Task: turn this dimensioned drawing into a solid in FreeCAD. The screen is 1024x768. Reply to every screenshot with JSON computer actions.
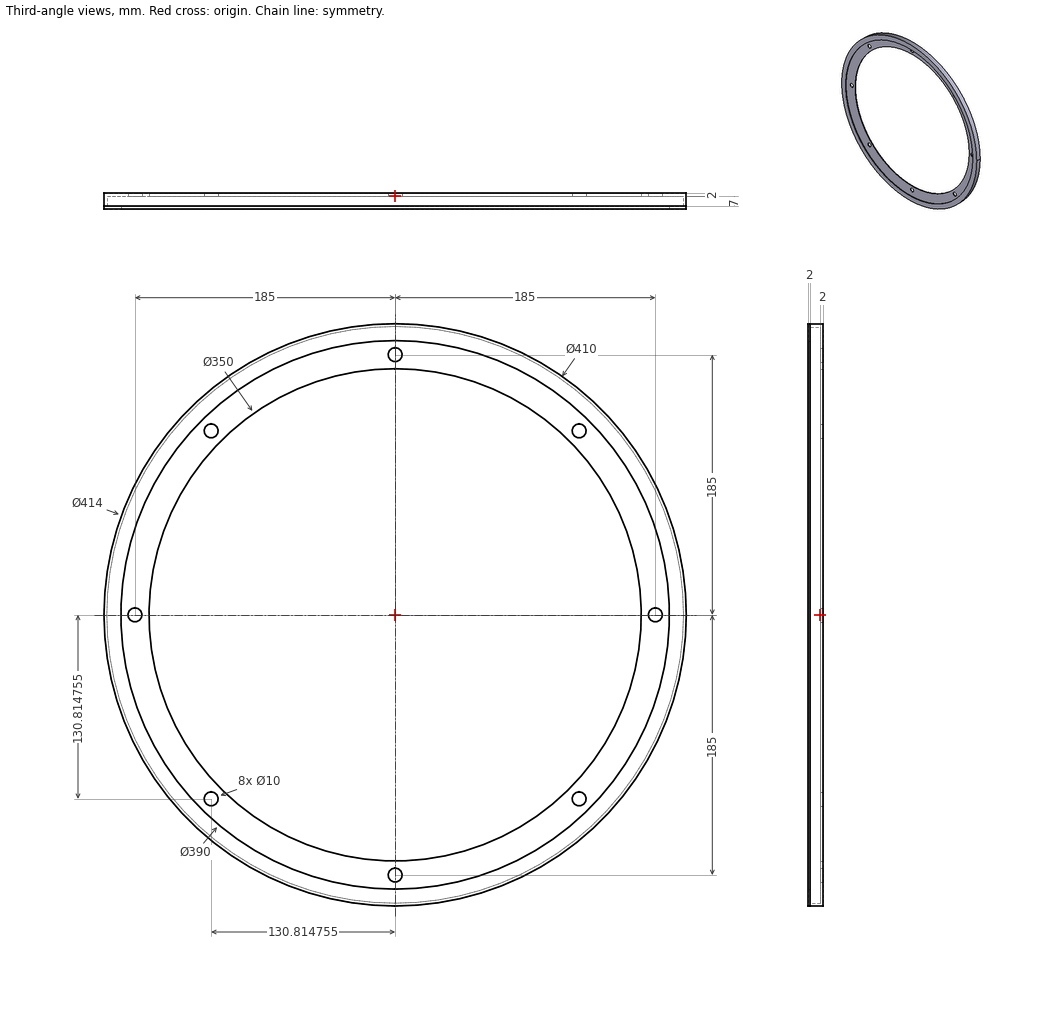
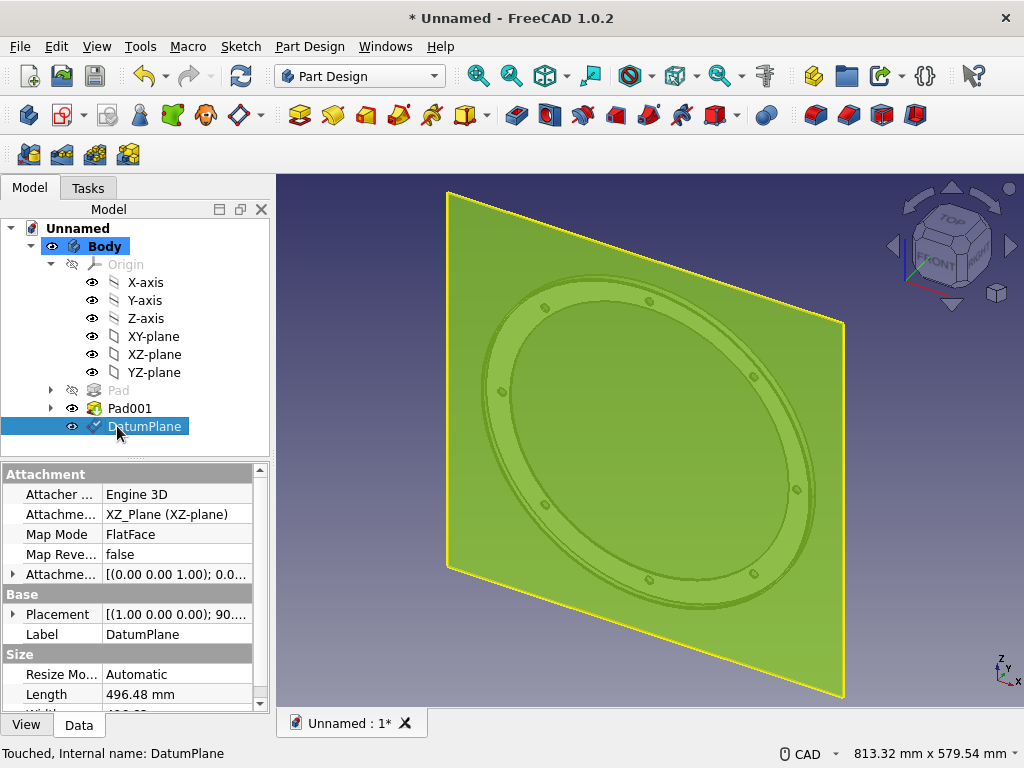
{"action": "left_click", "coordinate": [62, 116]}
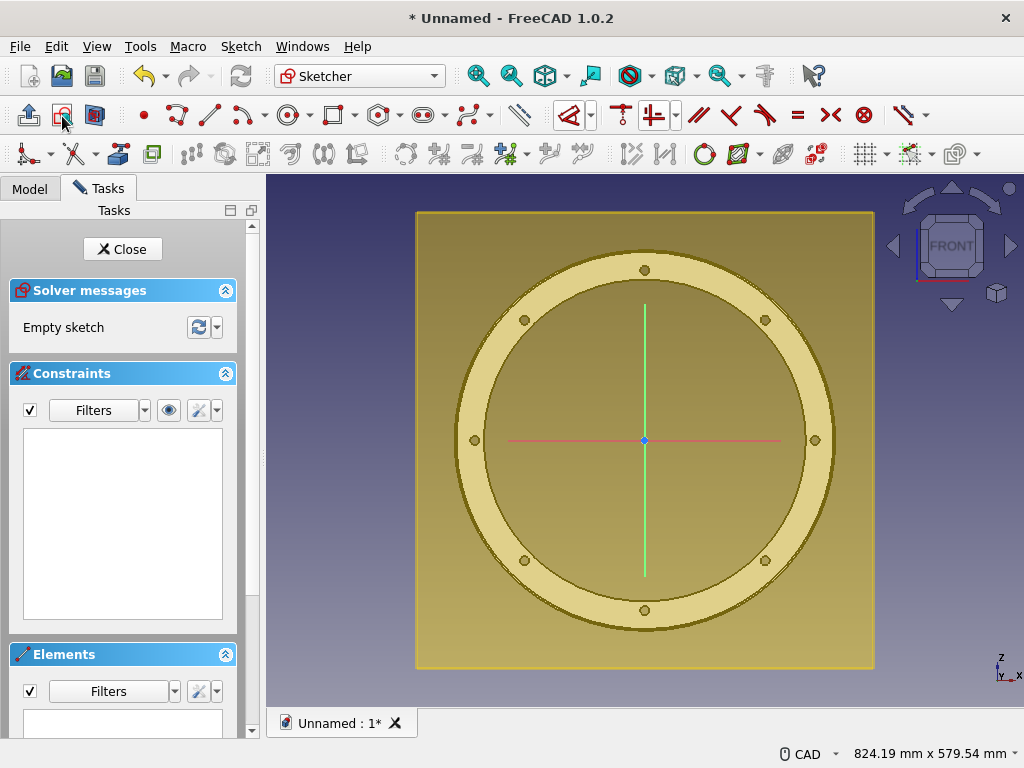
{"action": "scroll", "coordinate": [294, 440], "scroll_direction": "down", "scroll_amount": 1}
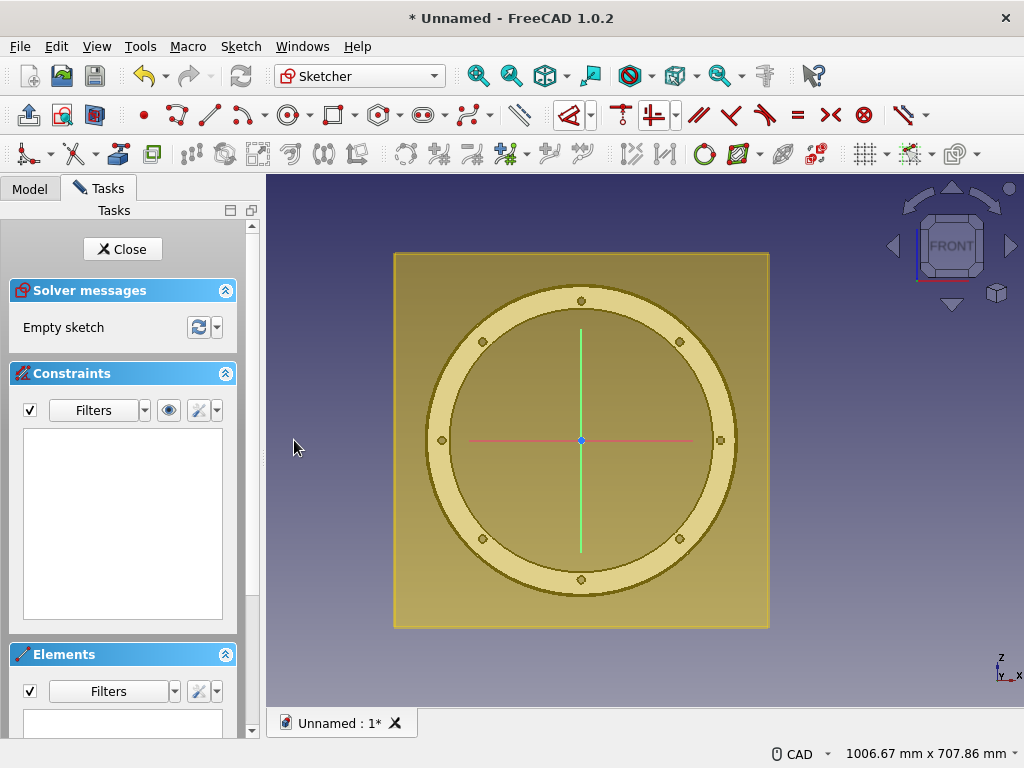
{"action": "left_click", "coordinate": [288, 116]}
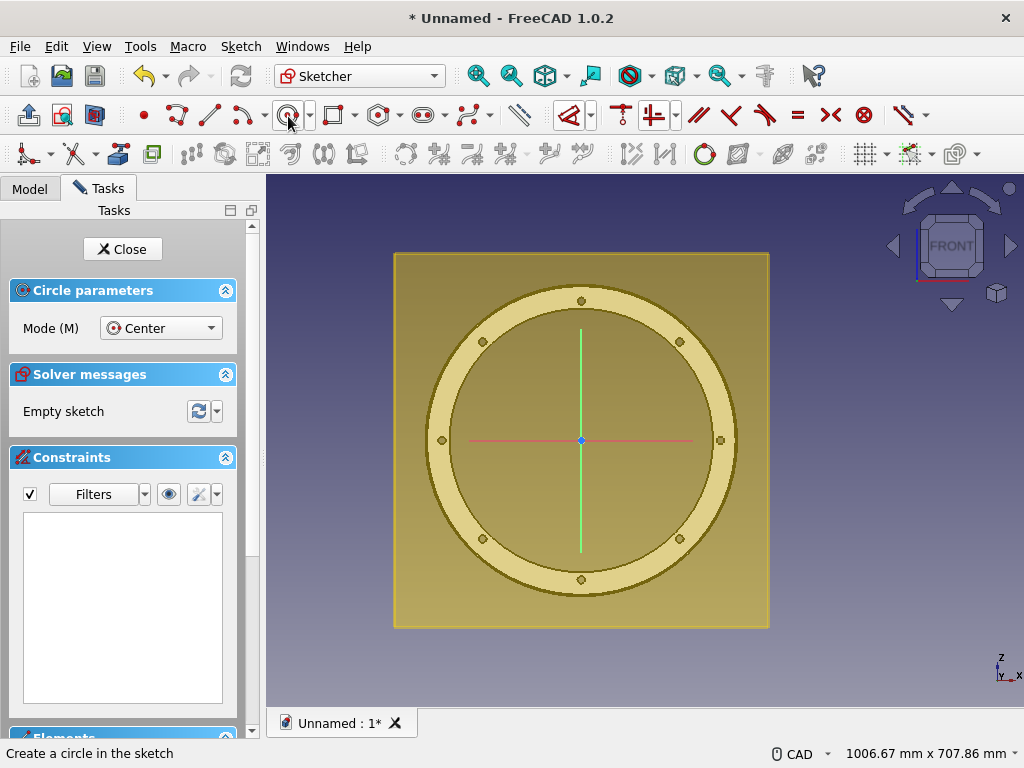
{"action": "left_click", "coordinate": [581, 441]}
{"action": "mouse_move", "coordinate": [691, 330]}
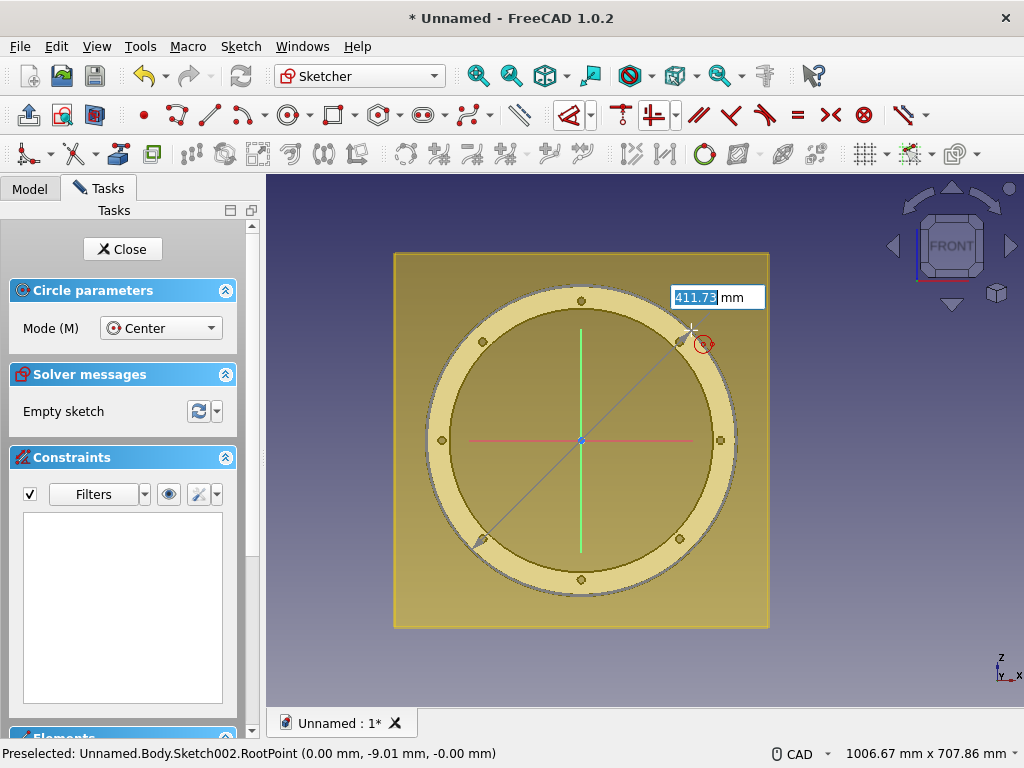
{"action": "type", "text": "414"}
{"action": "key", "text": "Return"}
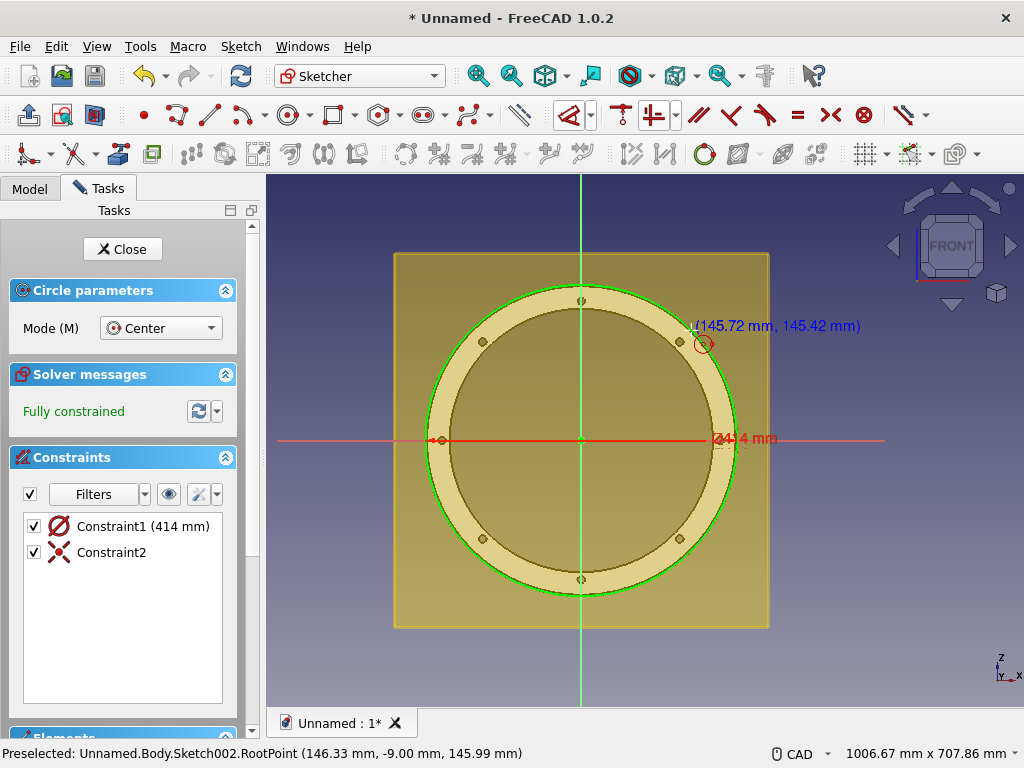
{"action": "left_click", "coordinate": [581, 441]}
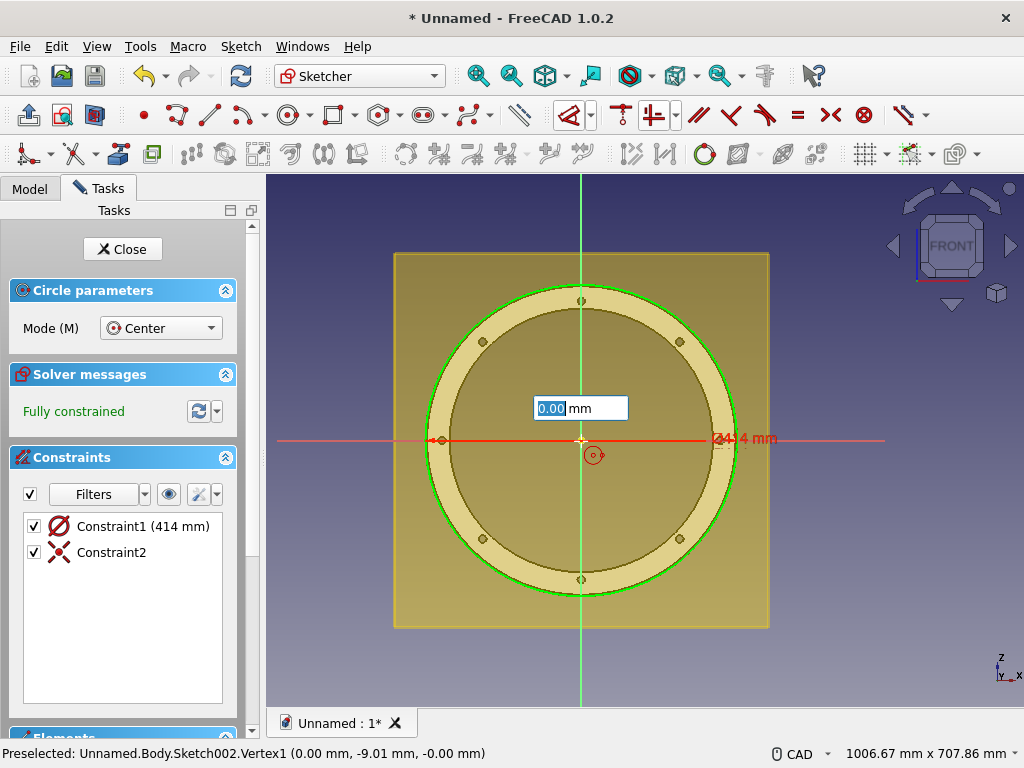
{"action": "scroll", "coordinate": [531, 578], "scroll_direction": "up", "scroll_amount": 3}
{"action": "mouse_move", "coordinate": [531, 578]}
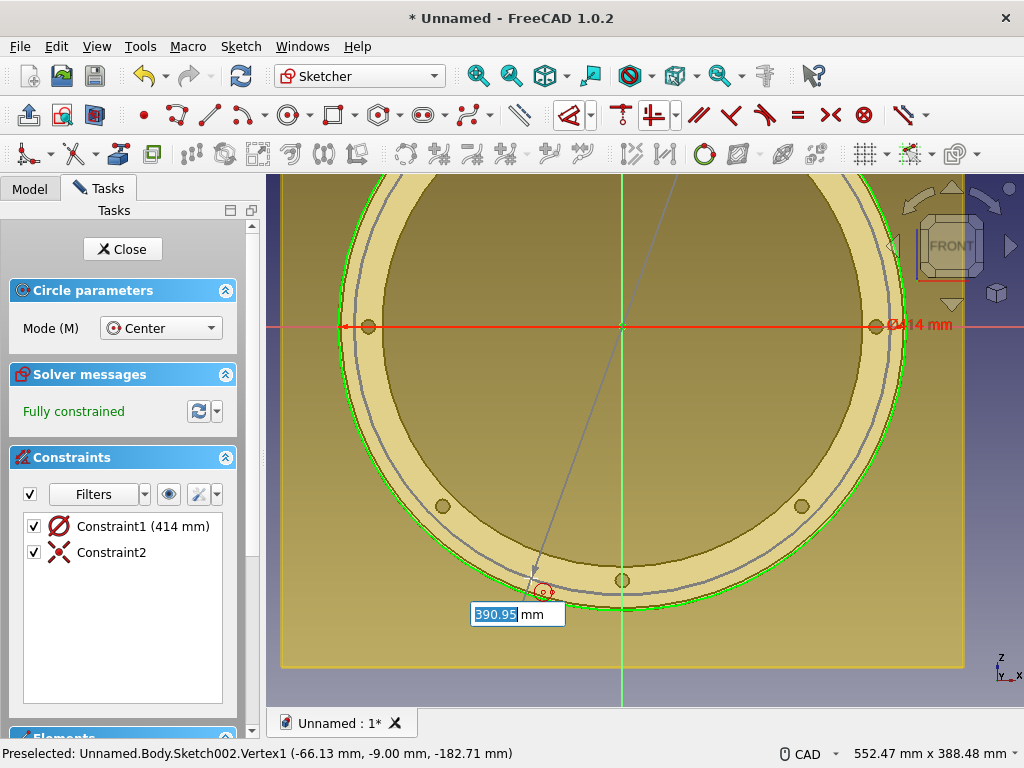
{"action": "type", "text": "390"}
{"action": "key", "text": "Return"}
{"action": "key", "text": "Escape"}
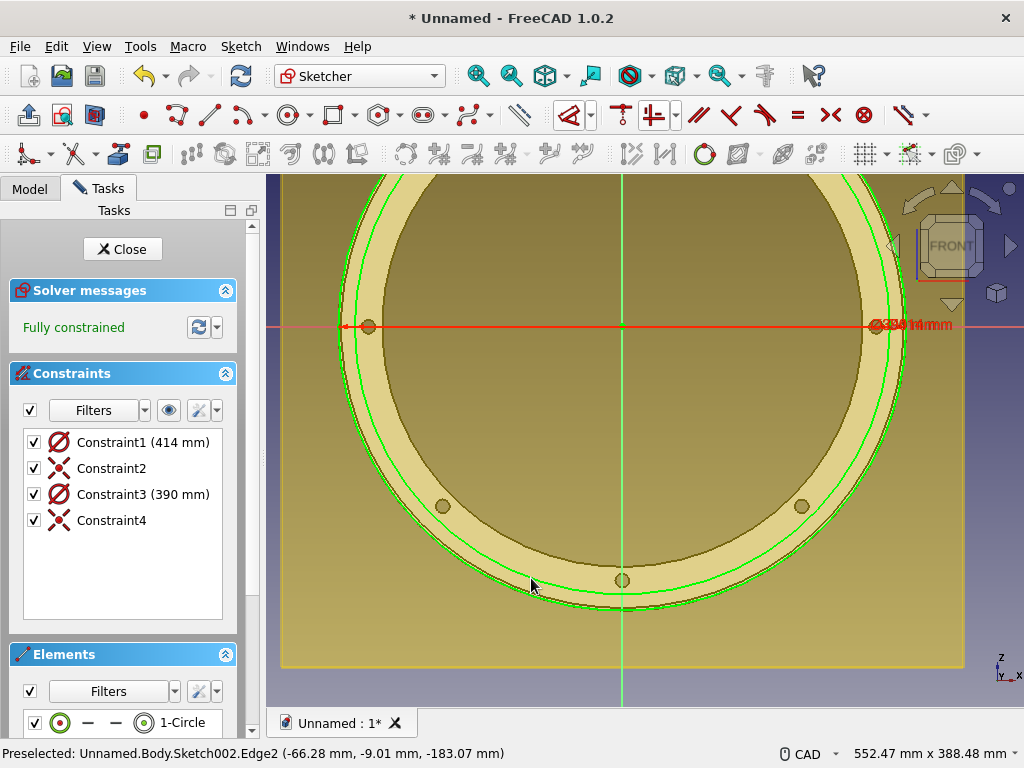
{"action": "left_click", "coordinate": [123, 249]}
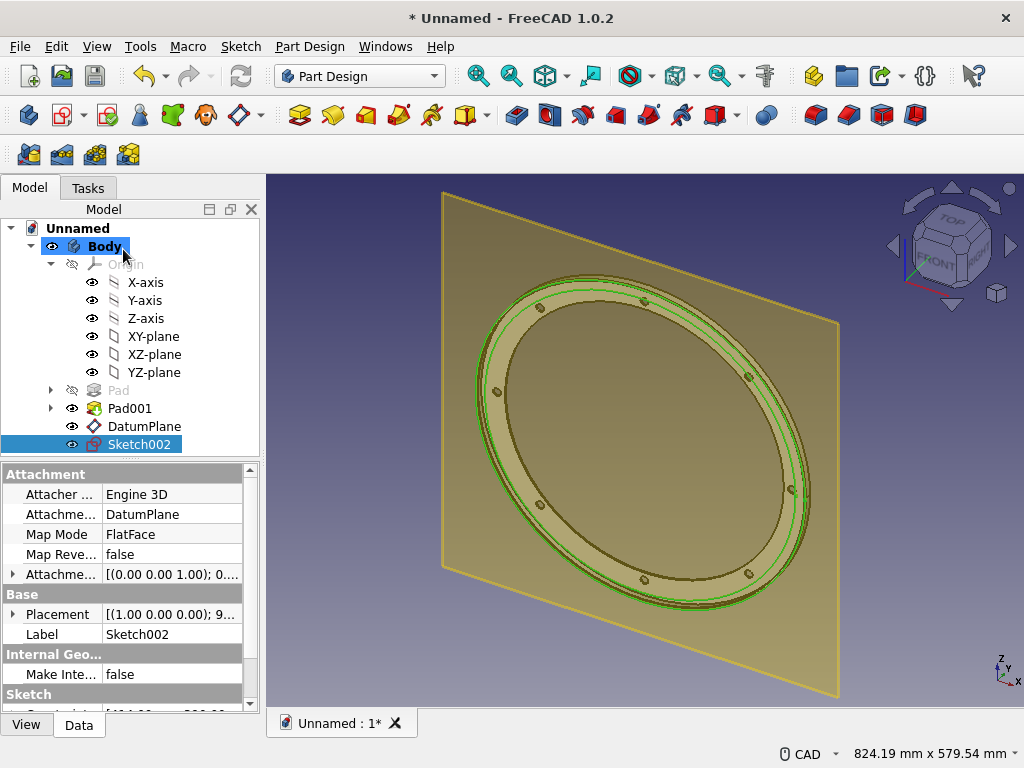
{"action": "left_click", "coordinate": [300, 116]}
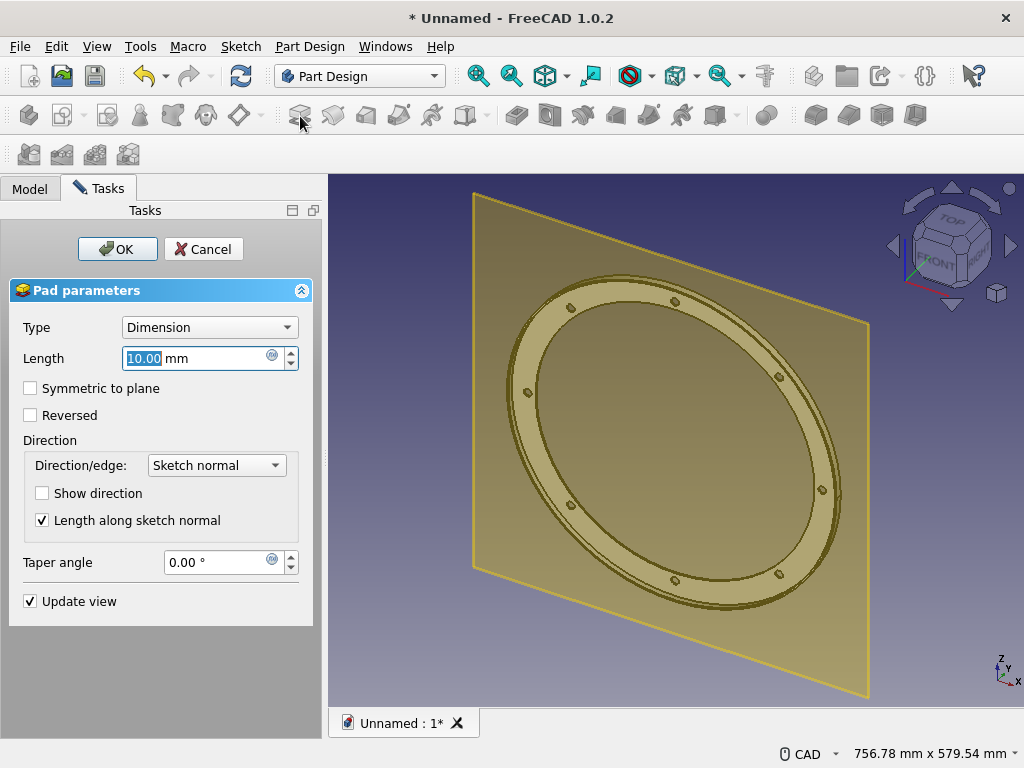
{"action": "type", "text": "2"}
{"action": "key", "text": "Tab"}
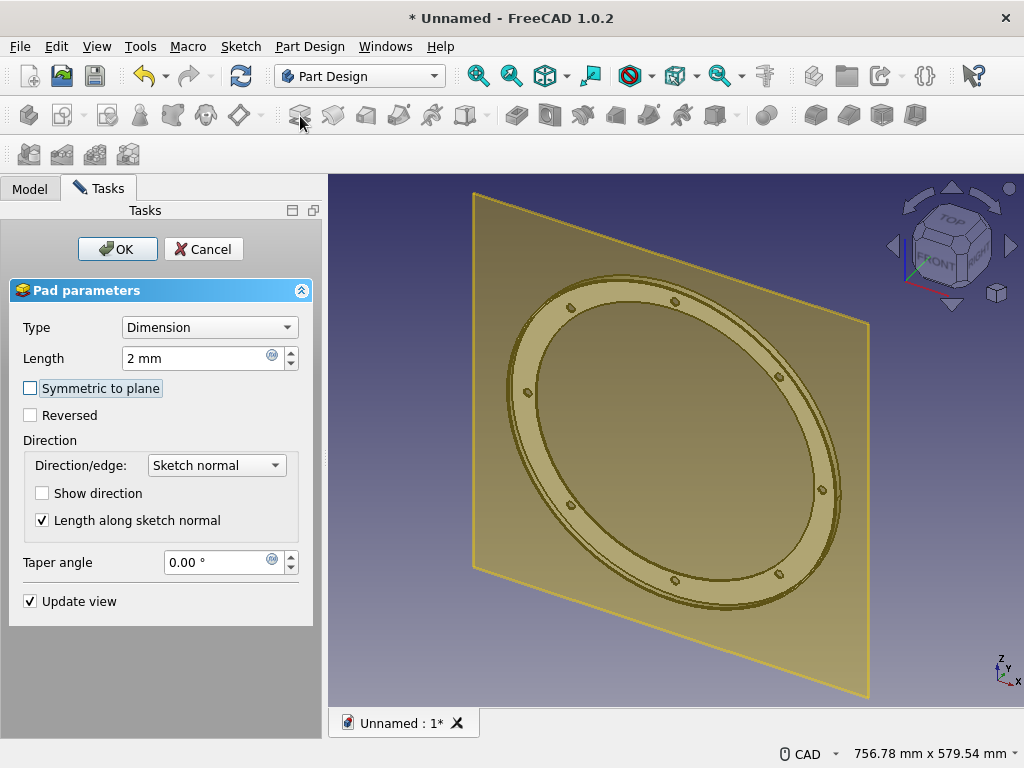
{"action": "left_click", "coordinate": [31, 415]}